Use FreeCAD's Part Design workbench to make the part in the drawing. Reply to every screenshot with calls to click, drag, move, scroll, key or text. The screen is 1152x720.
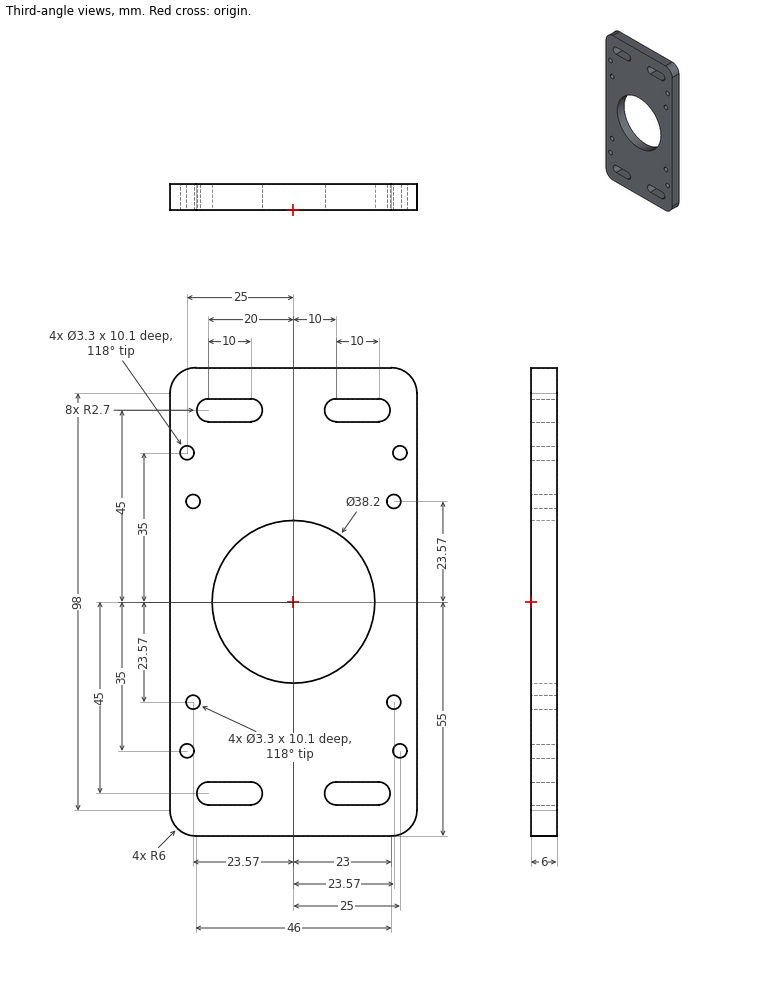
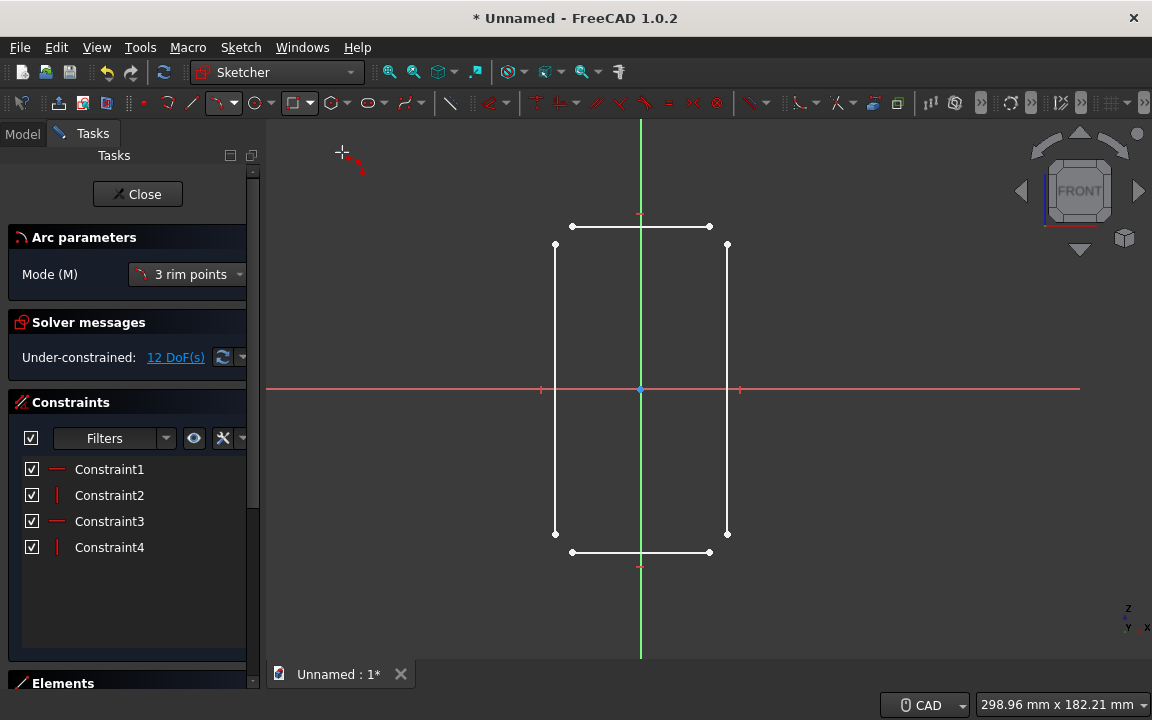
click(572, 553)
click(555, 535)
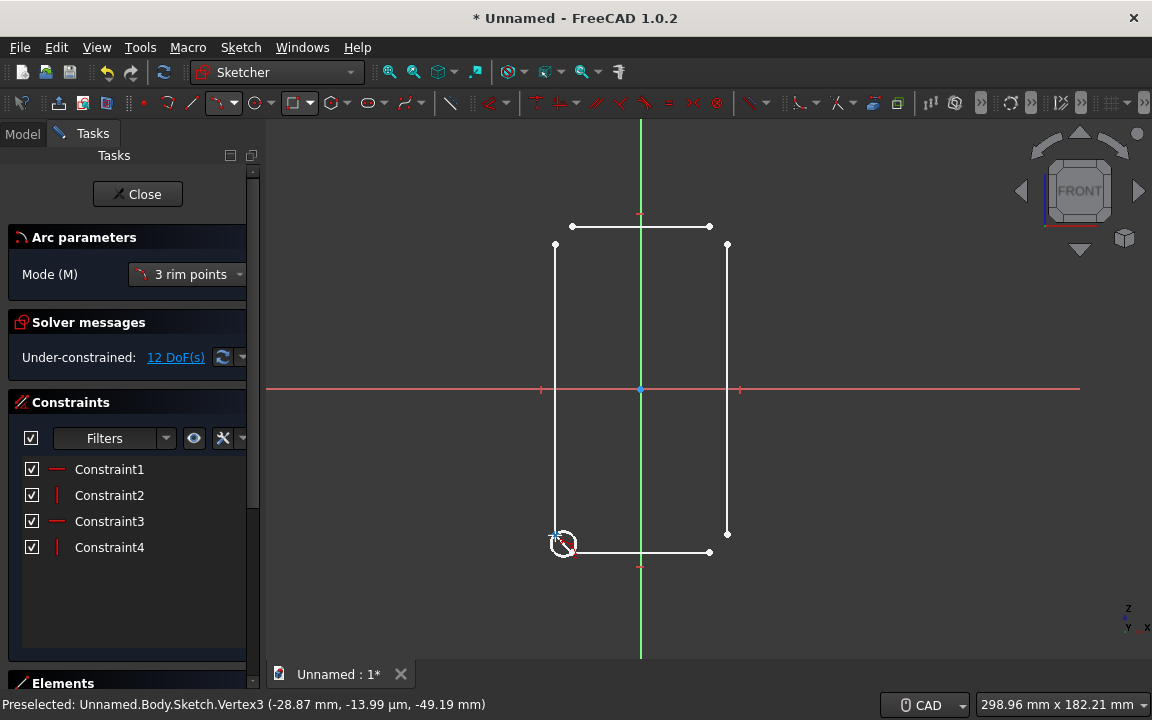
scroll(560, 547, up, 6)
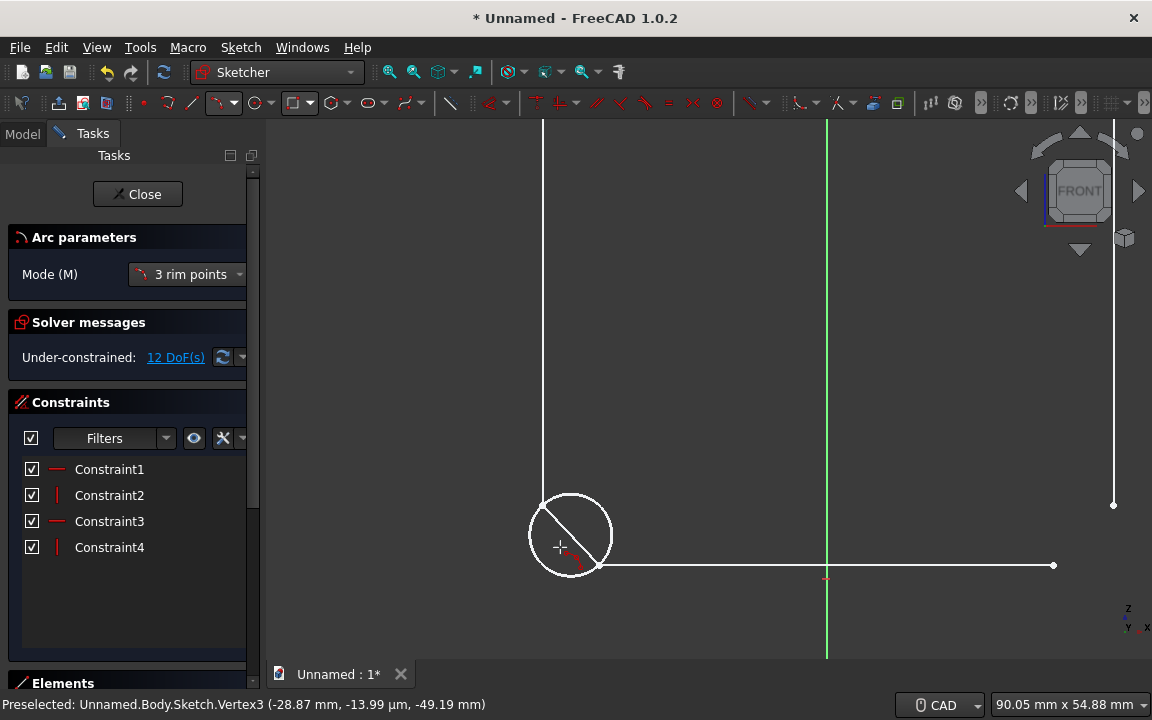
click(559, 545)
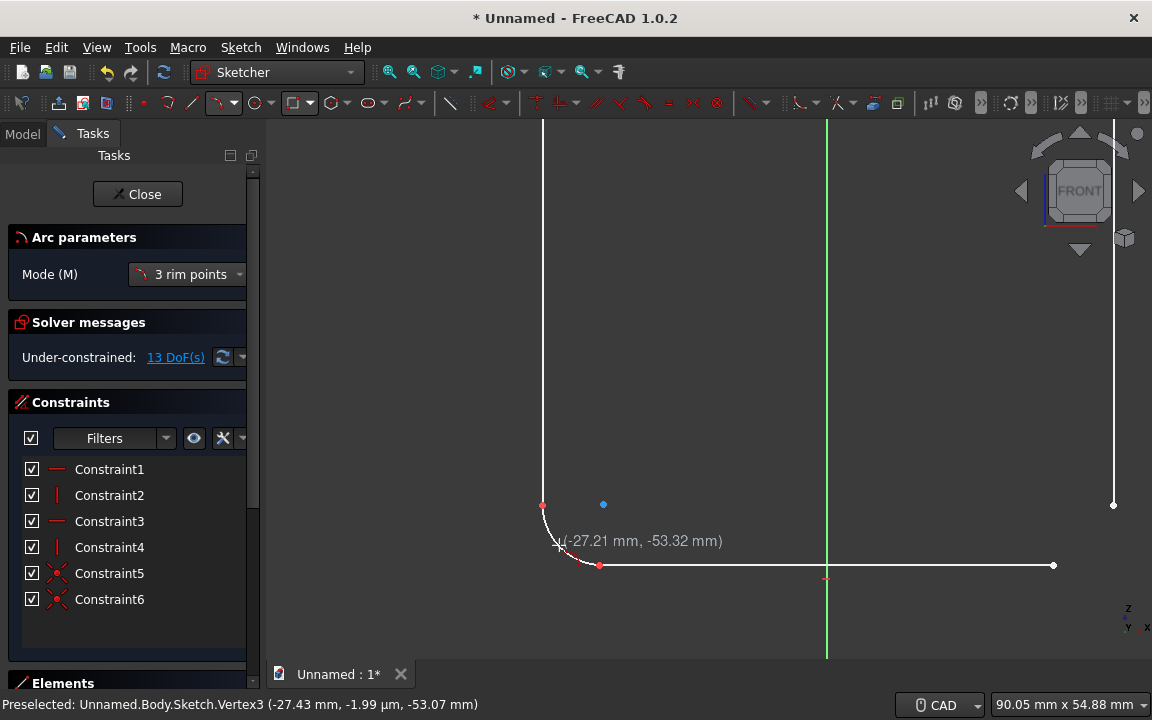
scroll(560, 547, down, 6)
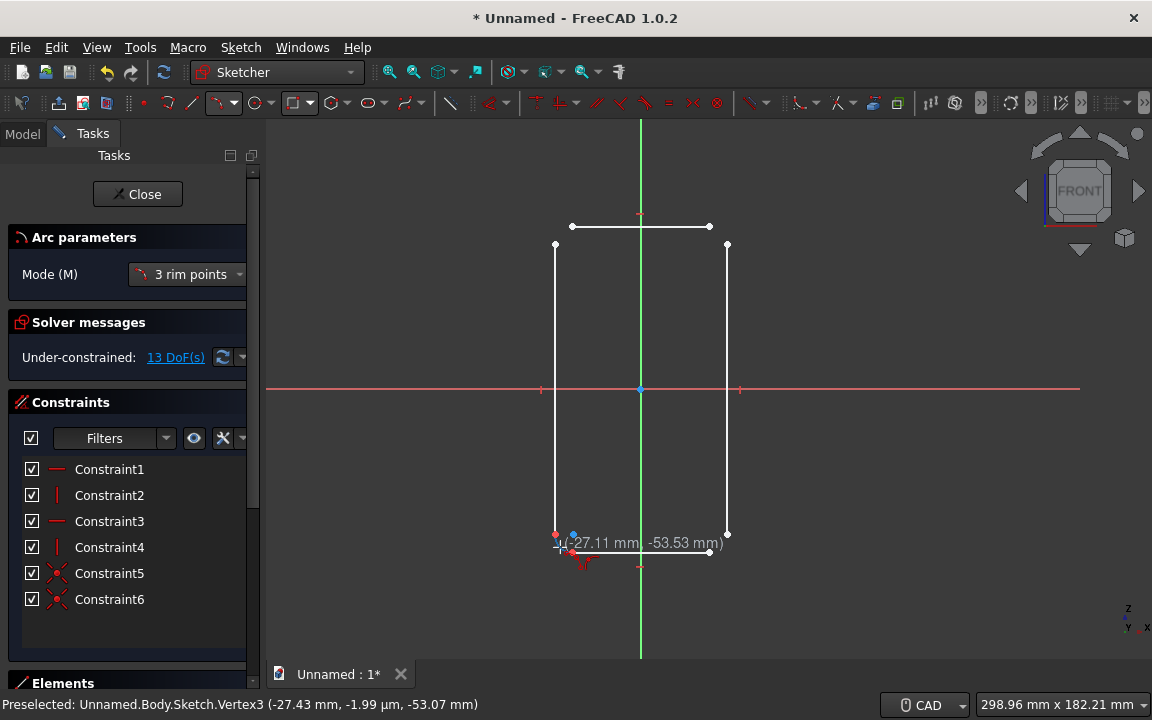
click(555, 245)
click(572, 227)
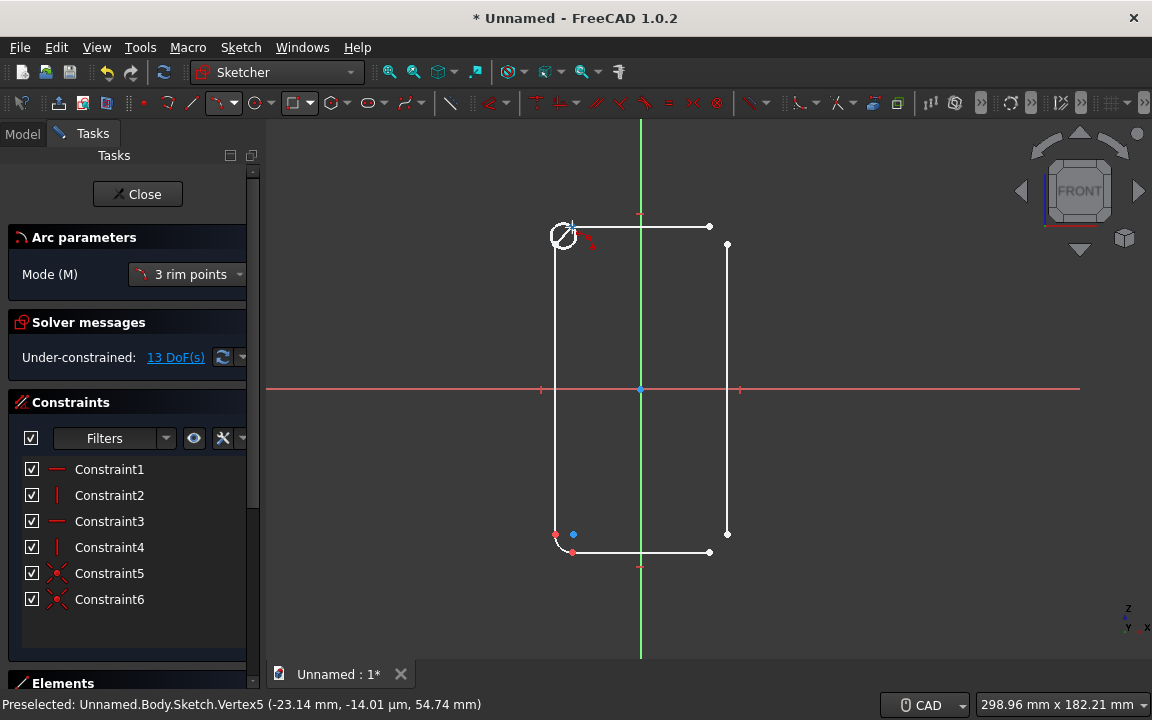
scroll(560, 231, up, 6)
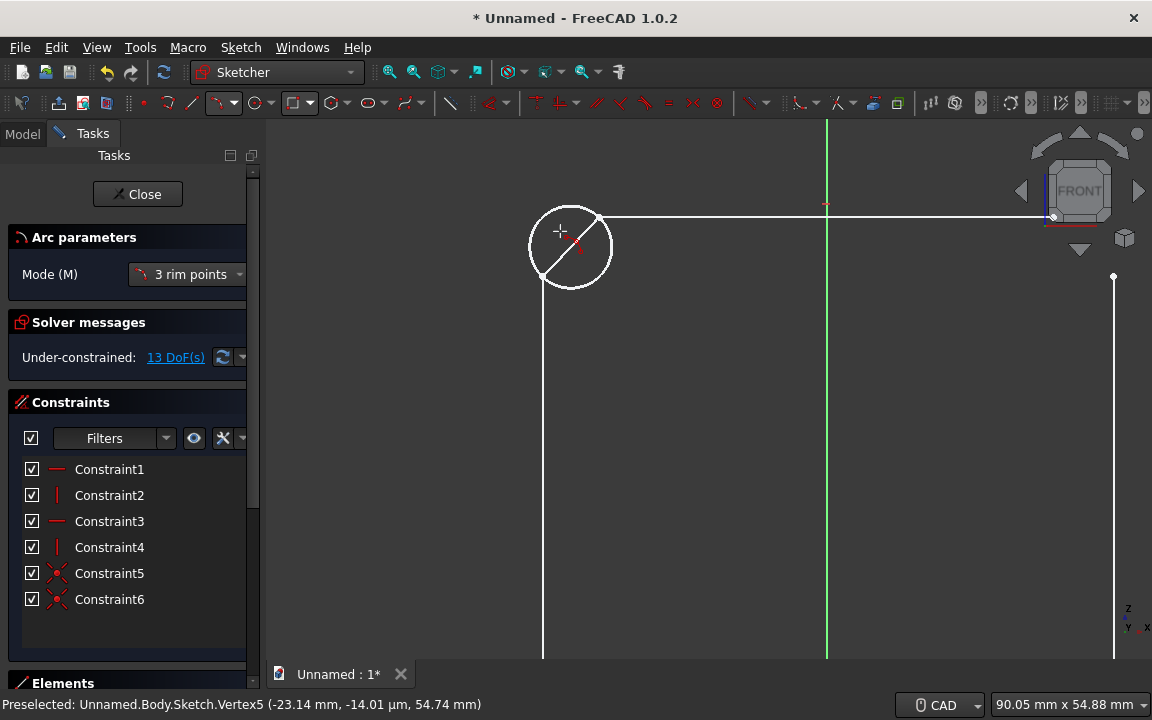
click(559, 232)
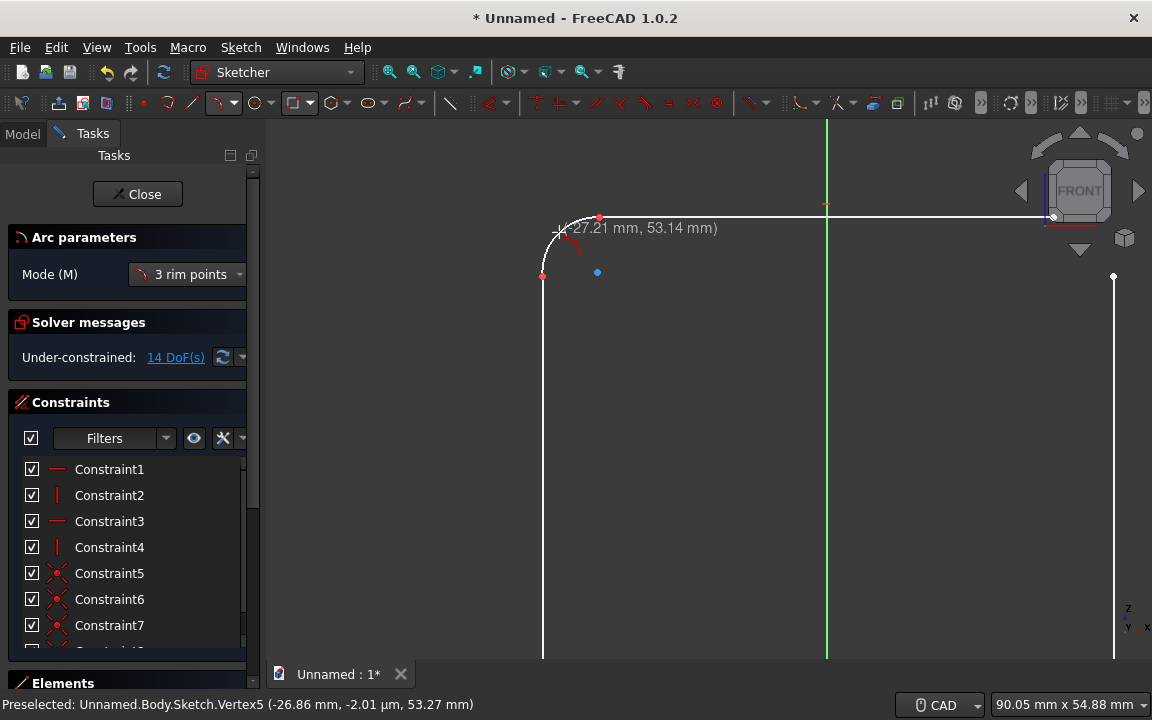
scroll(560, 231, down, 6)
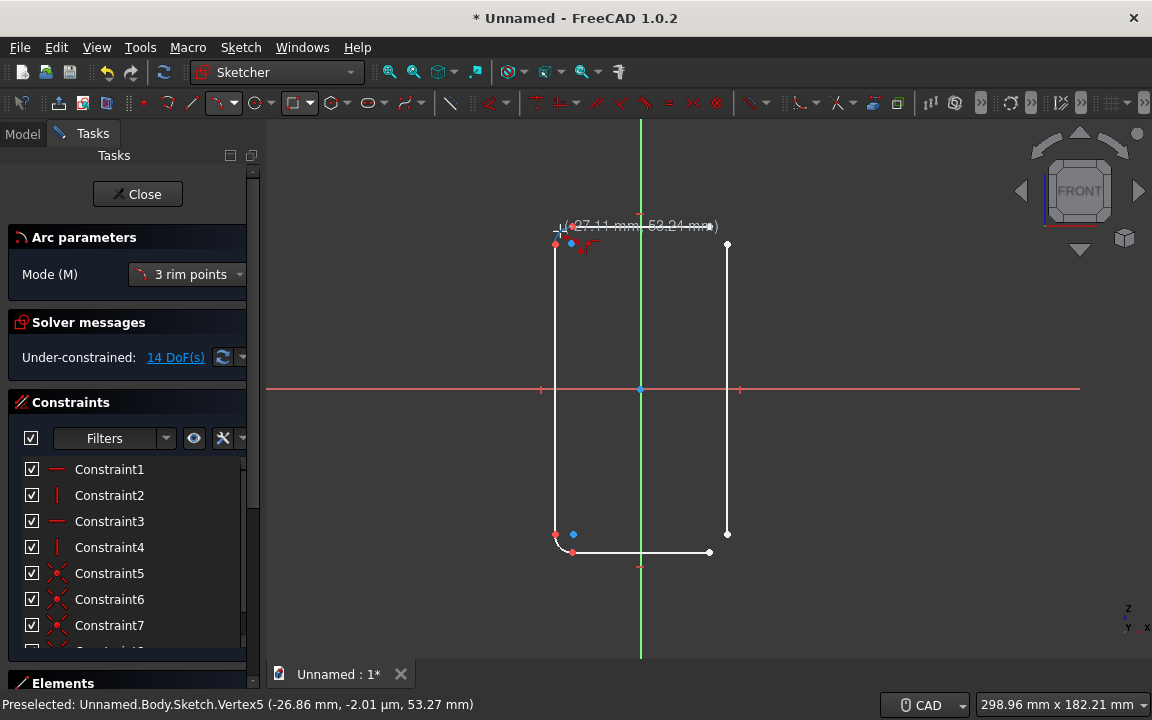
click(709, 227)
click(727, 245)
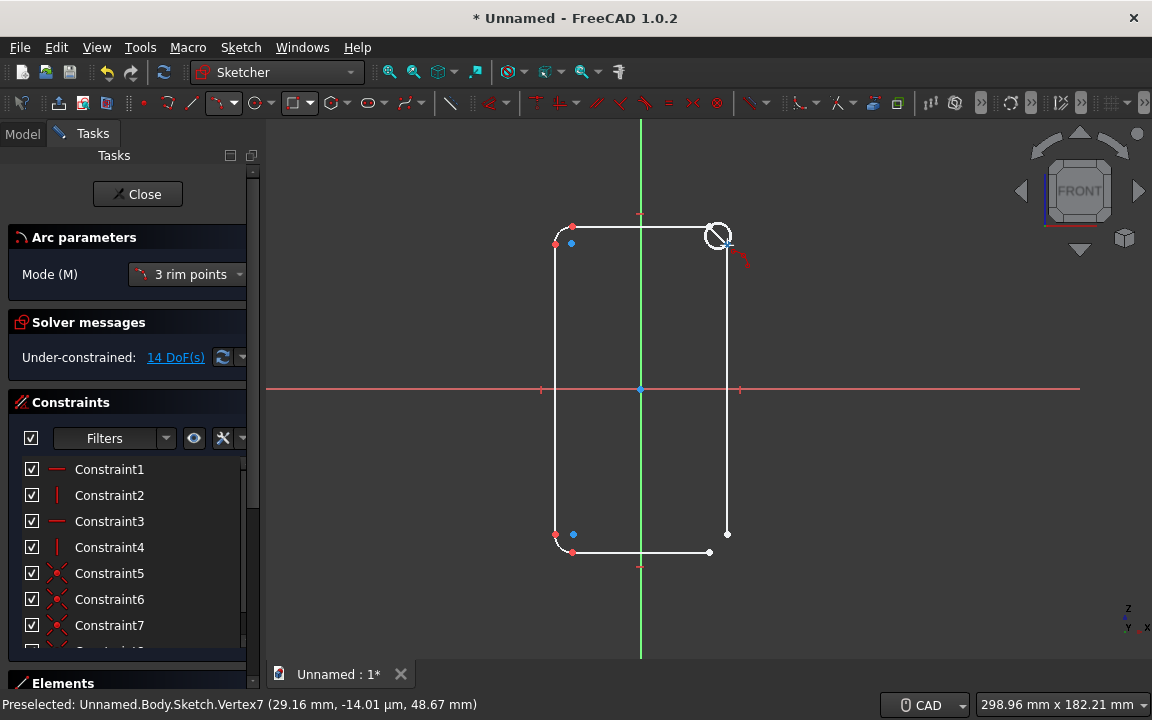
scroll(721, 231, up, 6)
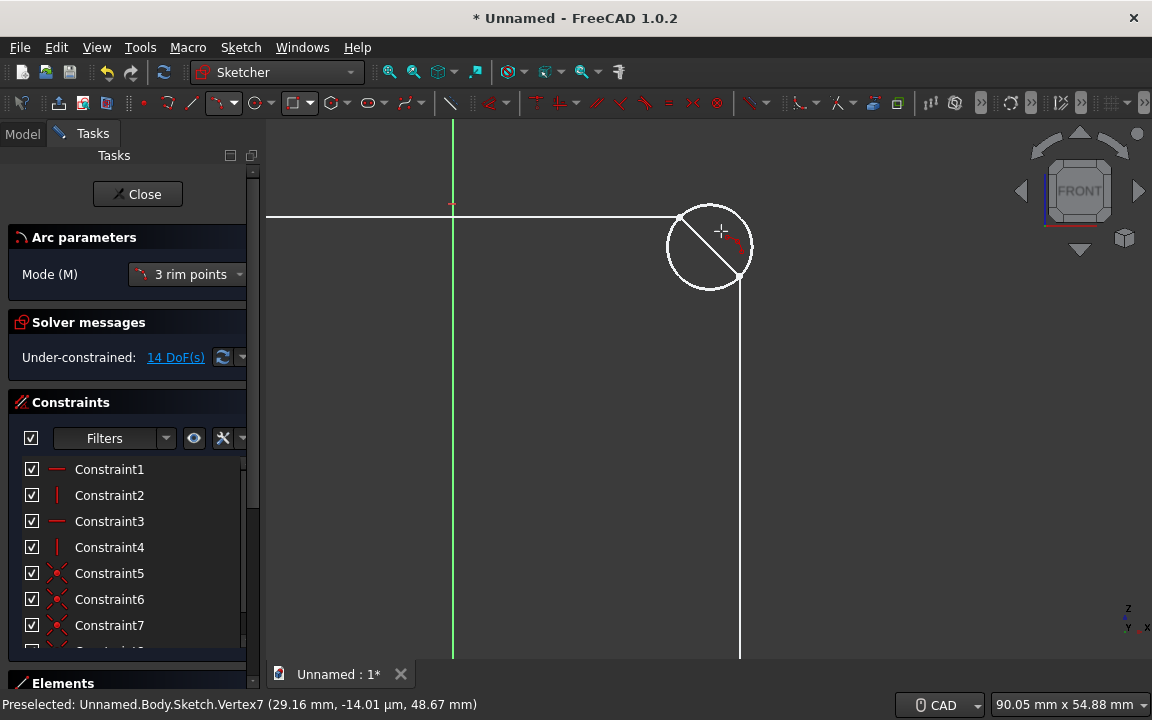
click(721, 232)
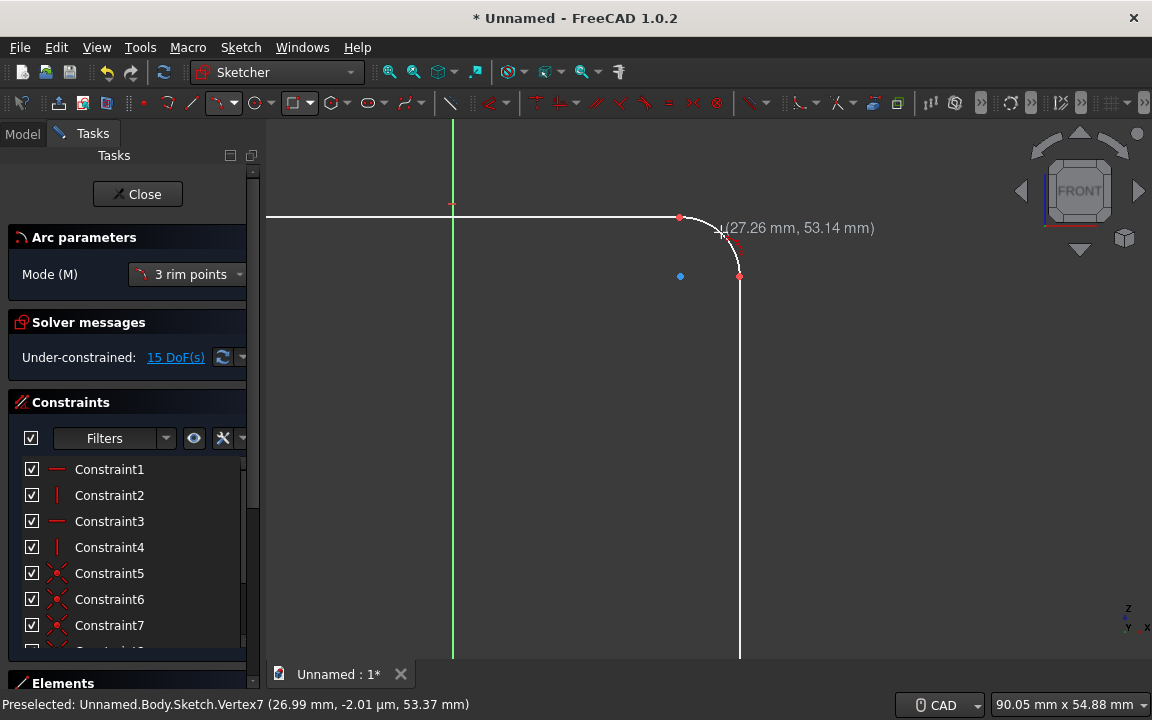
scroll(721, 231, down, 6)